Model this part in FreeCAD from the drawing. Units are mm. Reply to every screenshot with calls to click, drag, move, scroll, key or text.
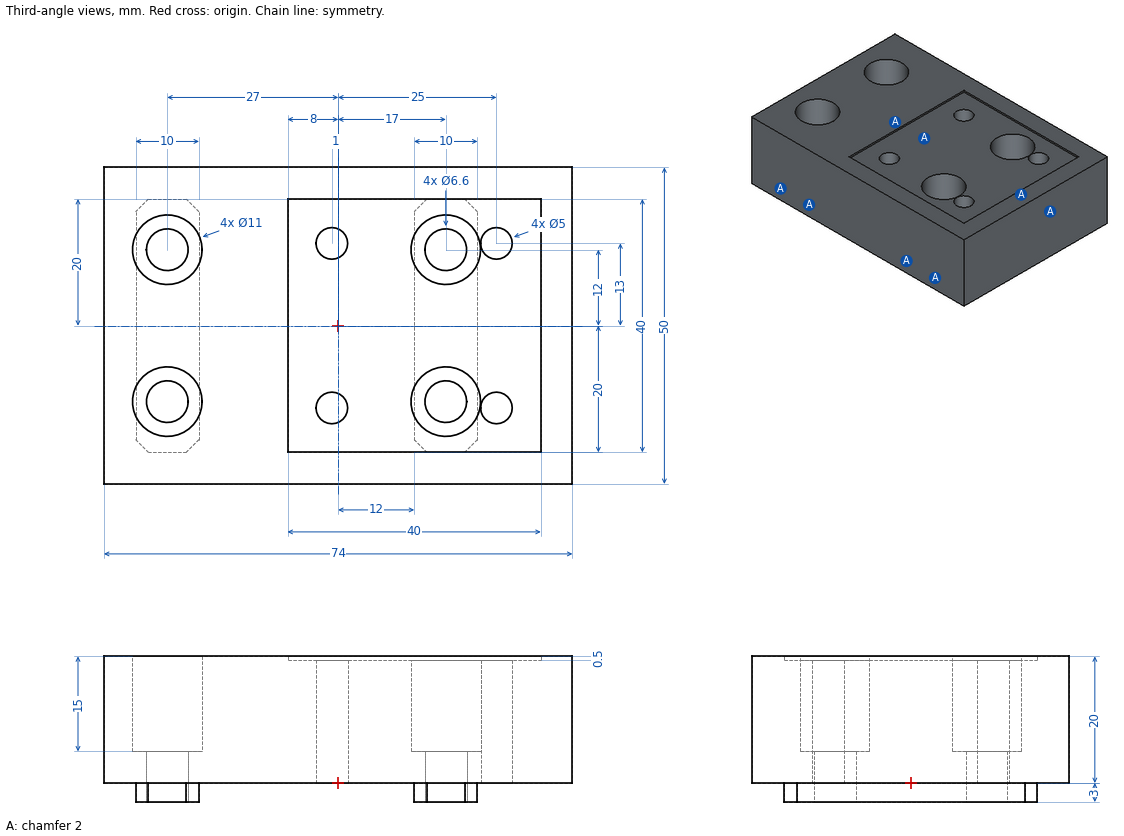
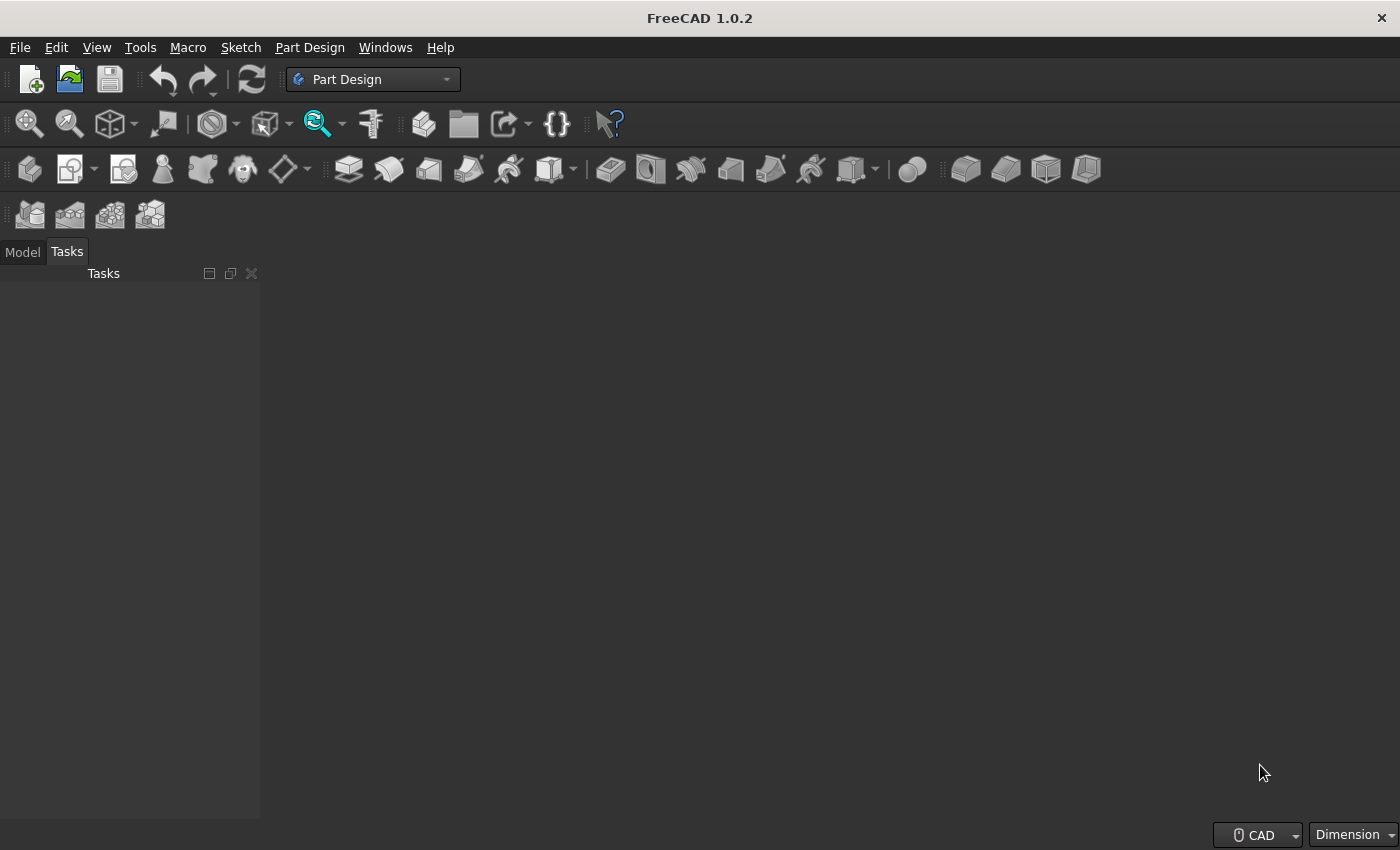
click(30, 80)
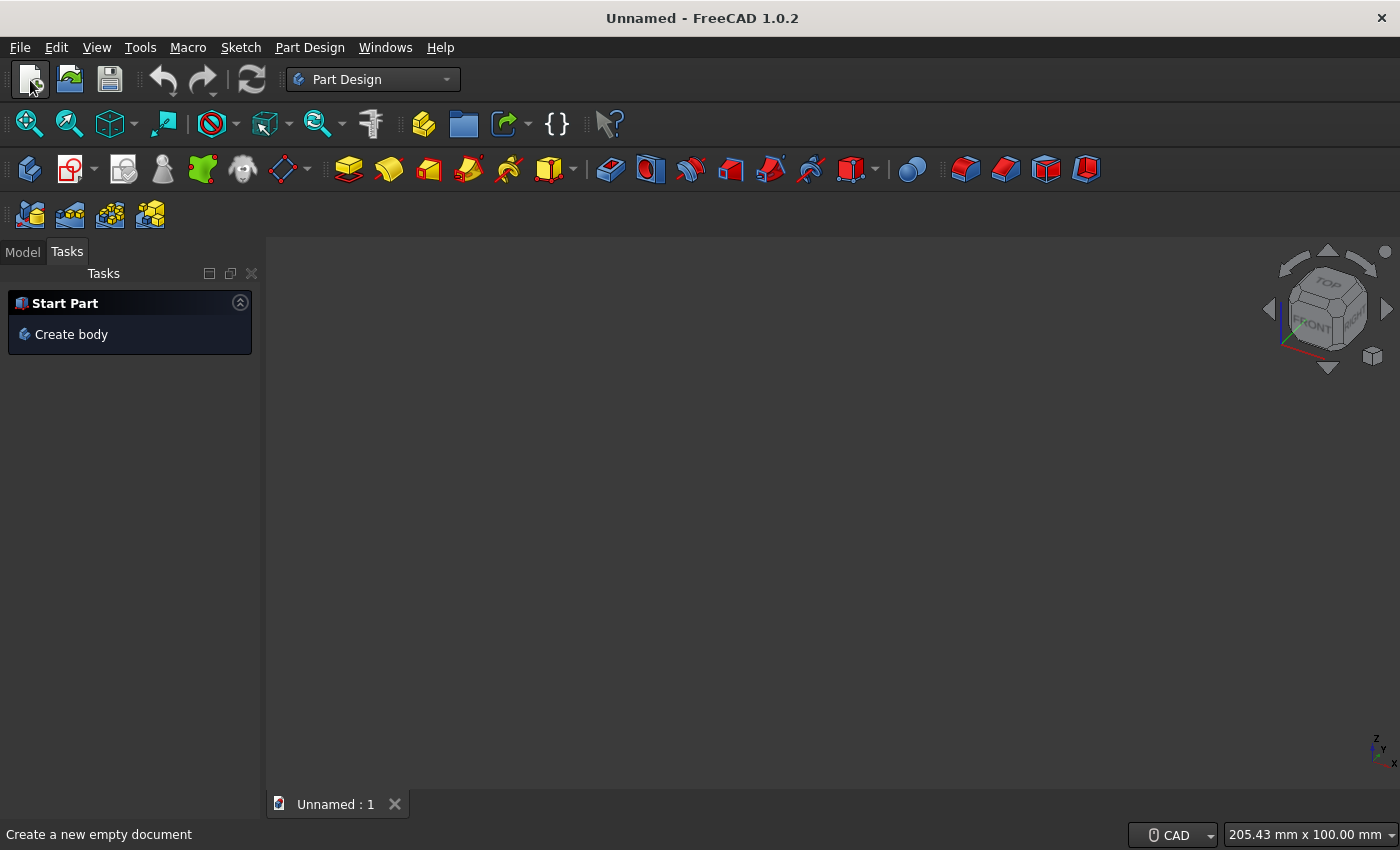
click(70, 170)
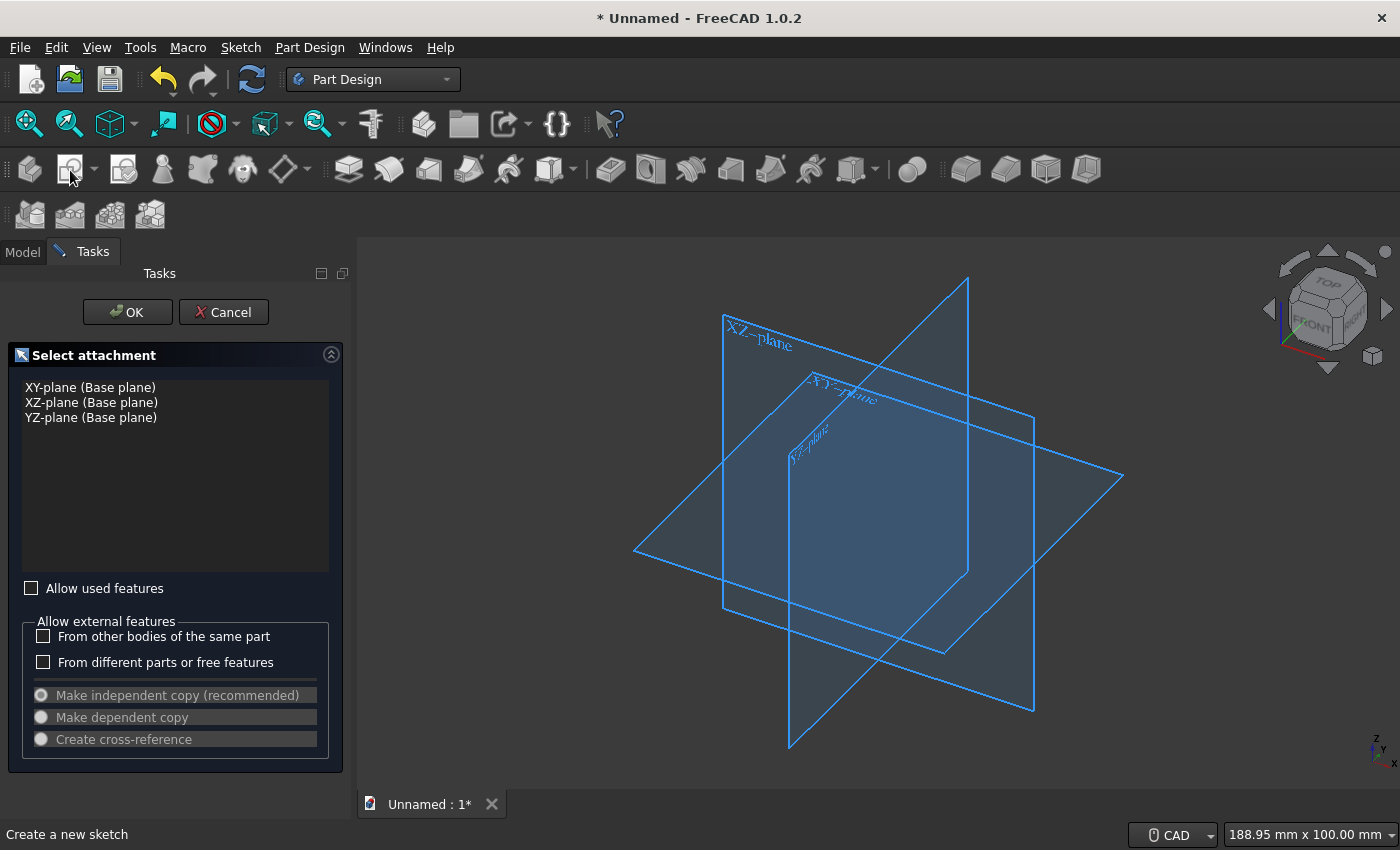
click(82, 388)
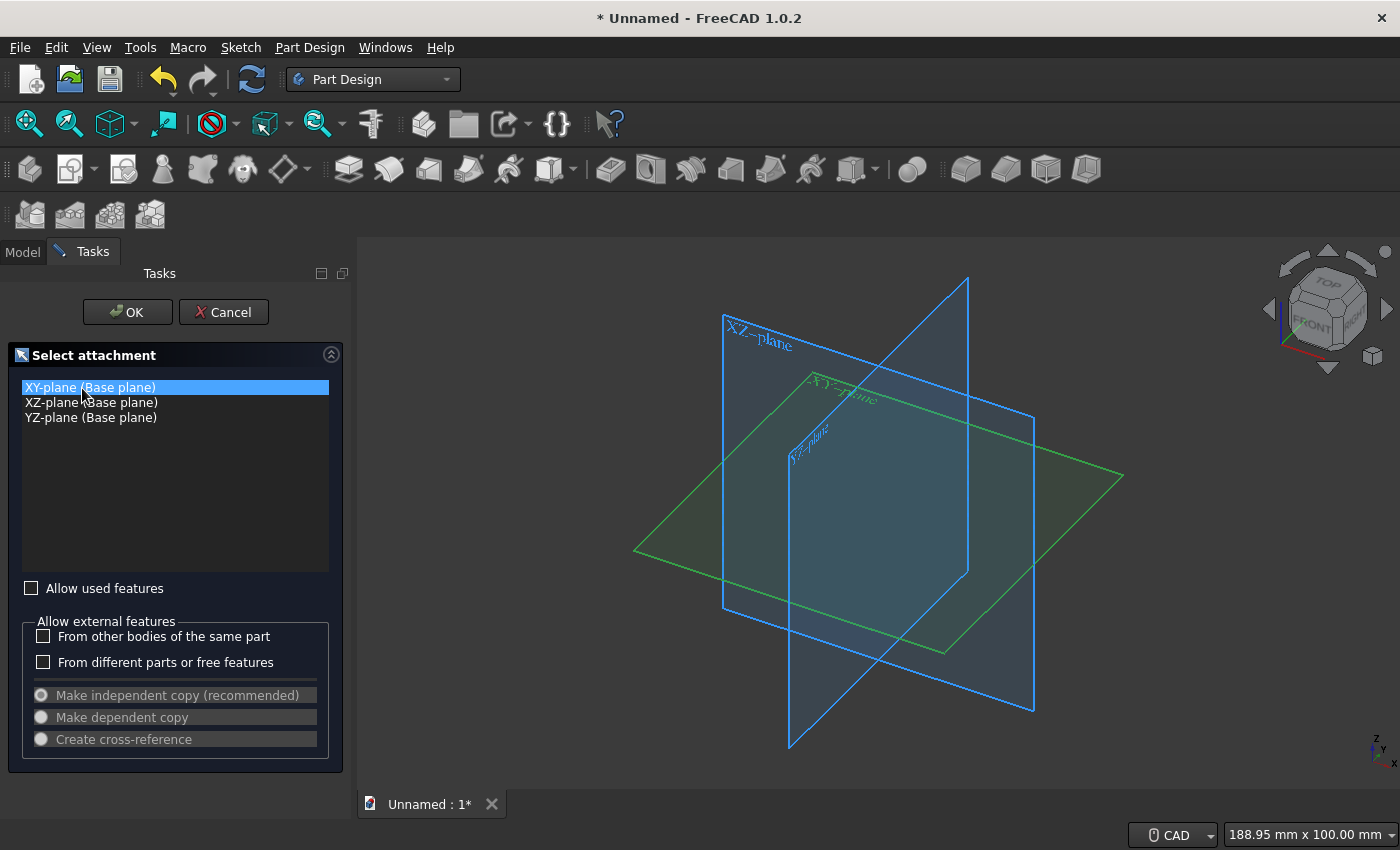
click(128, 312)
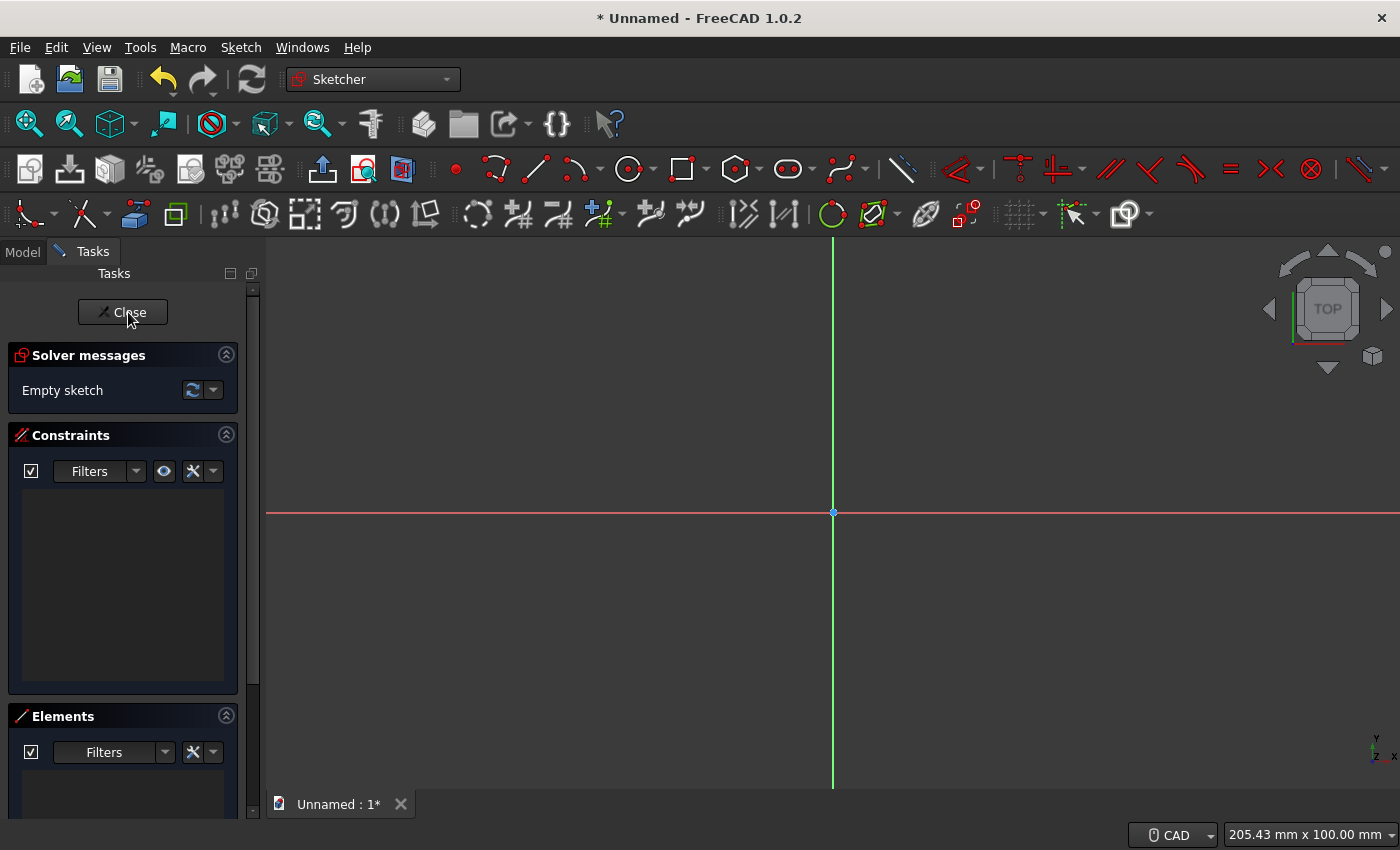
click(708, 170)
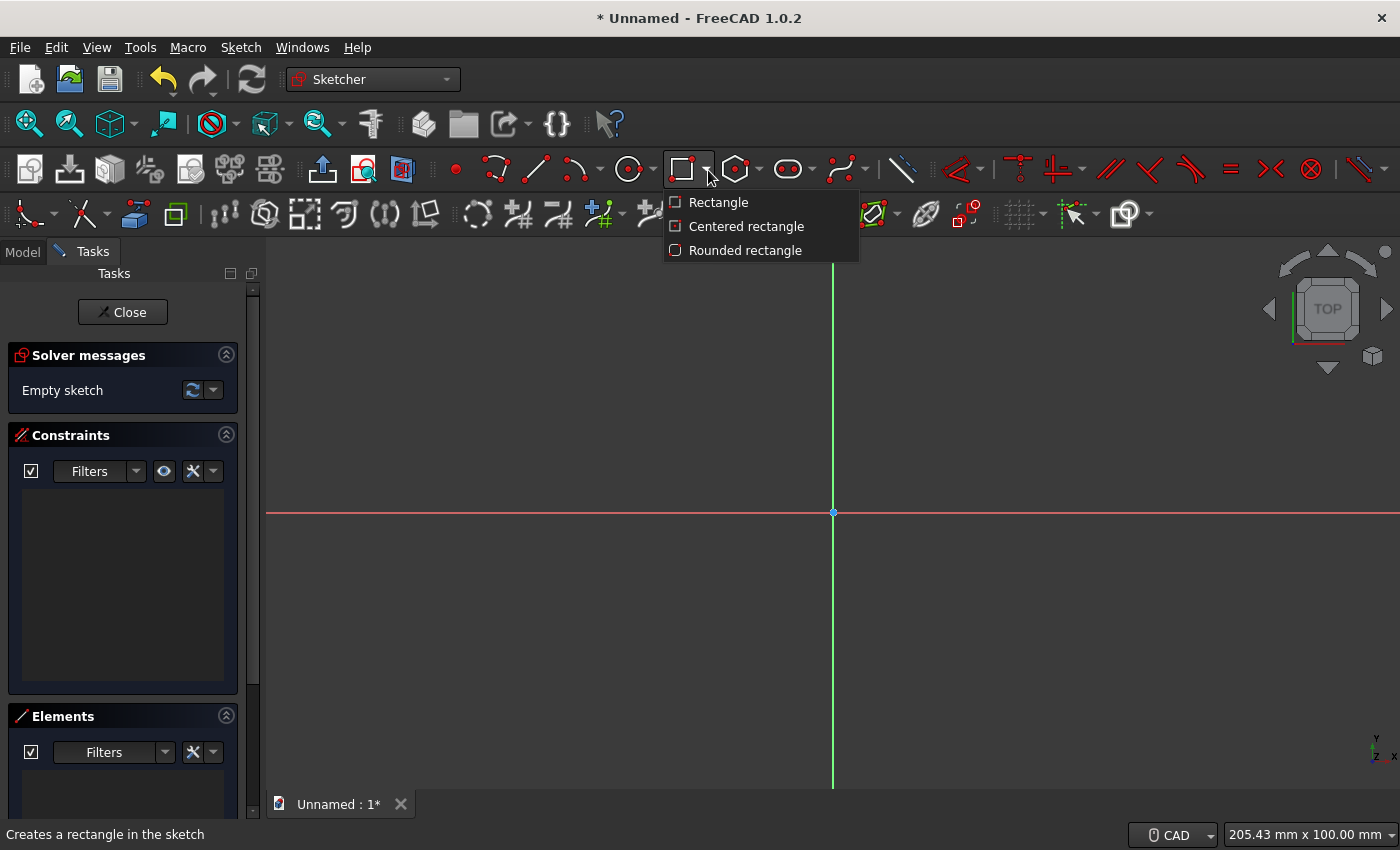
click(762, 226)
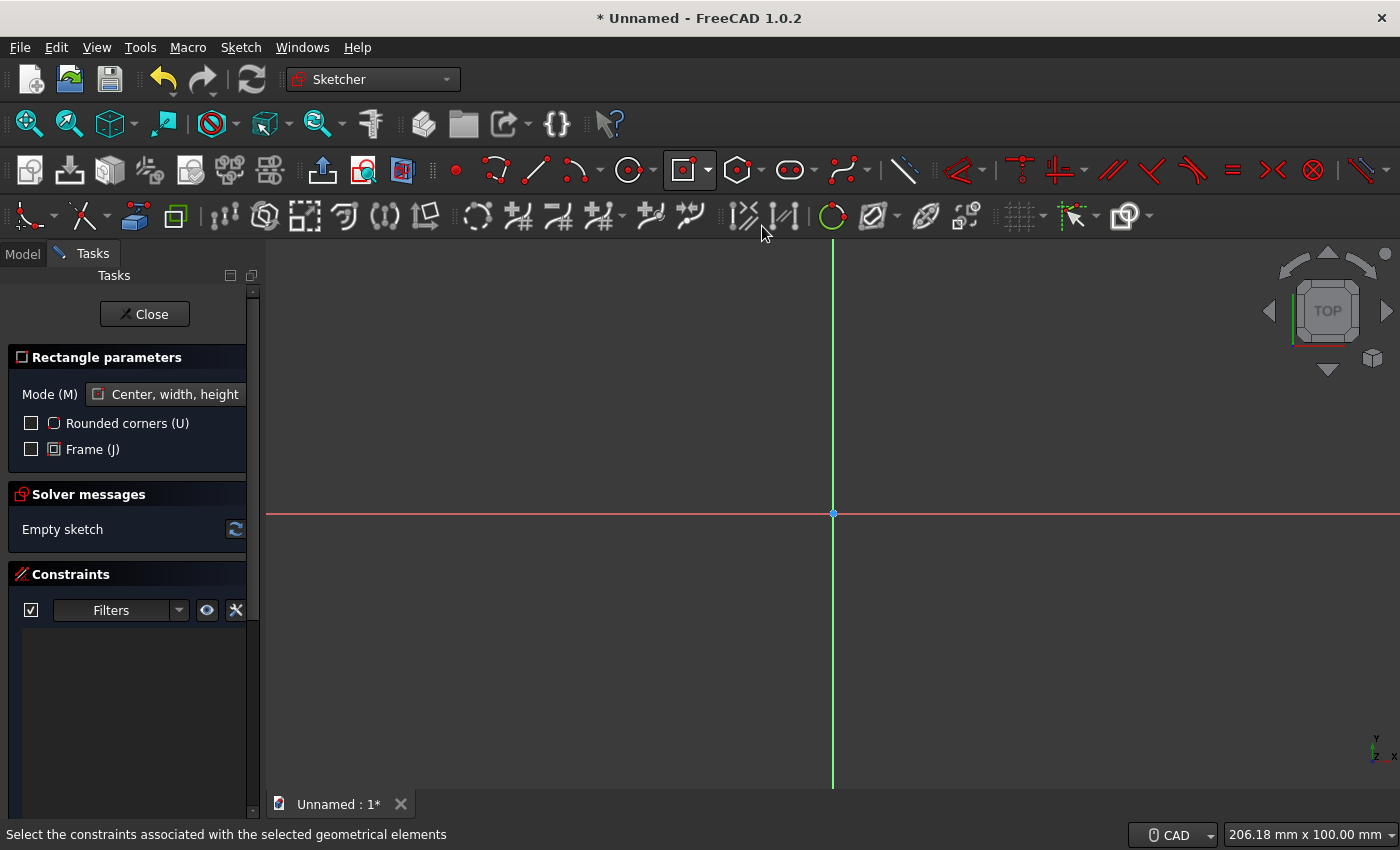
click(833, 514)
move(1036, 376)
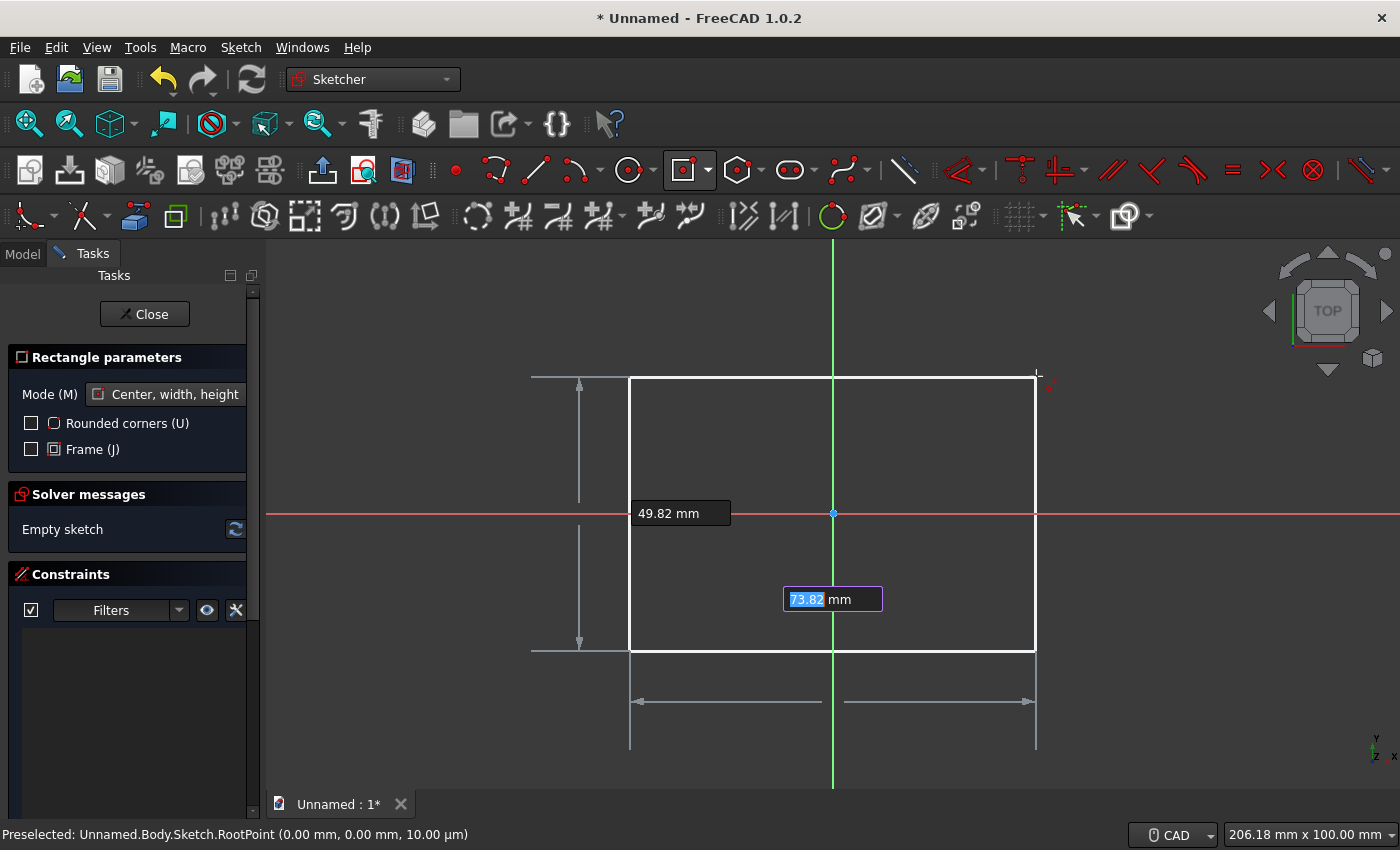
text(74)
key(Tab)
text(50)
key(Return)
key(Escape)